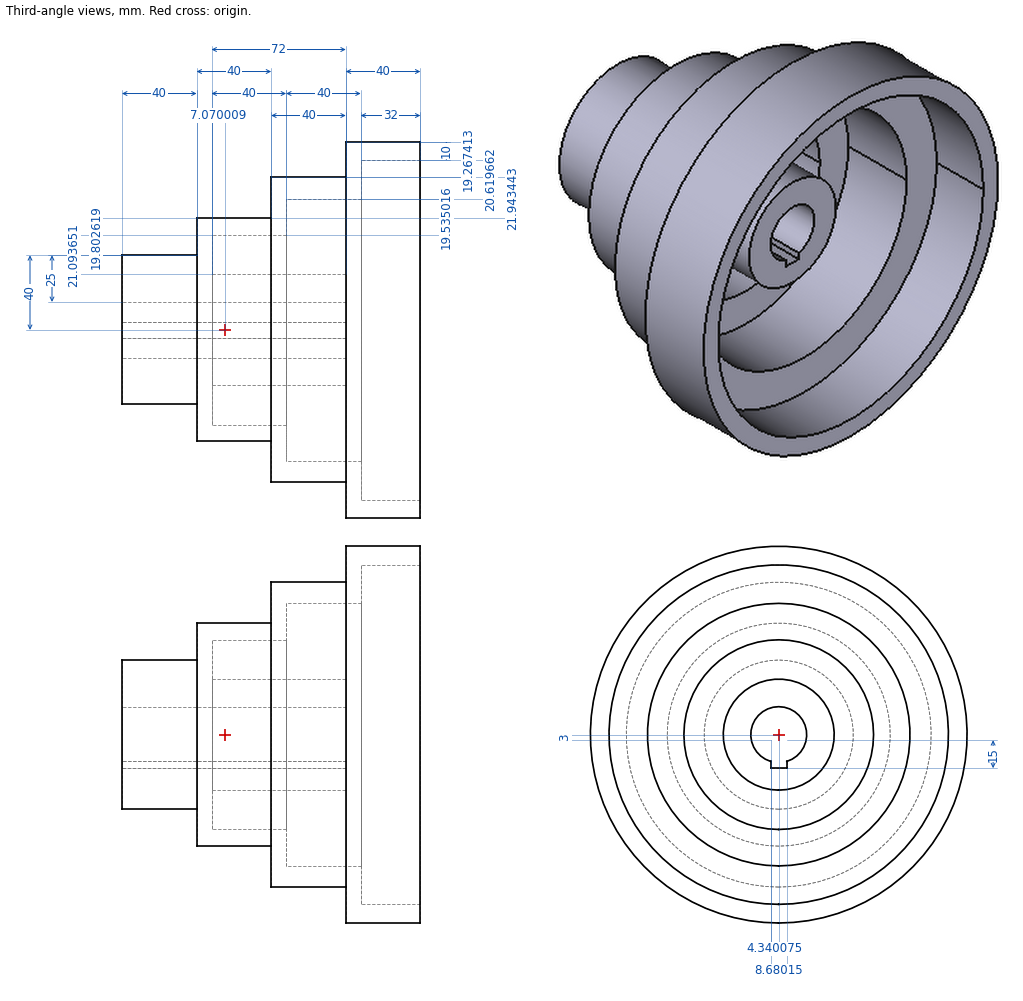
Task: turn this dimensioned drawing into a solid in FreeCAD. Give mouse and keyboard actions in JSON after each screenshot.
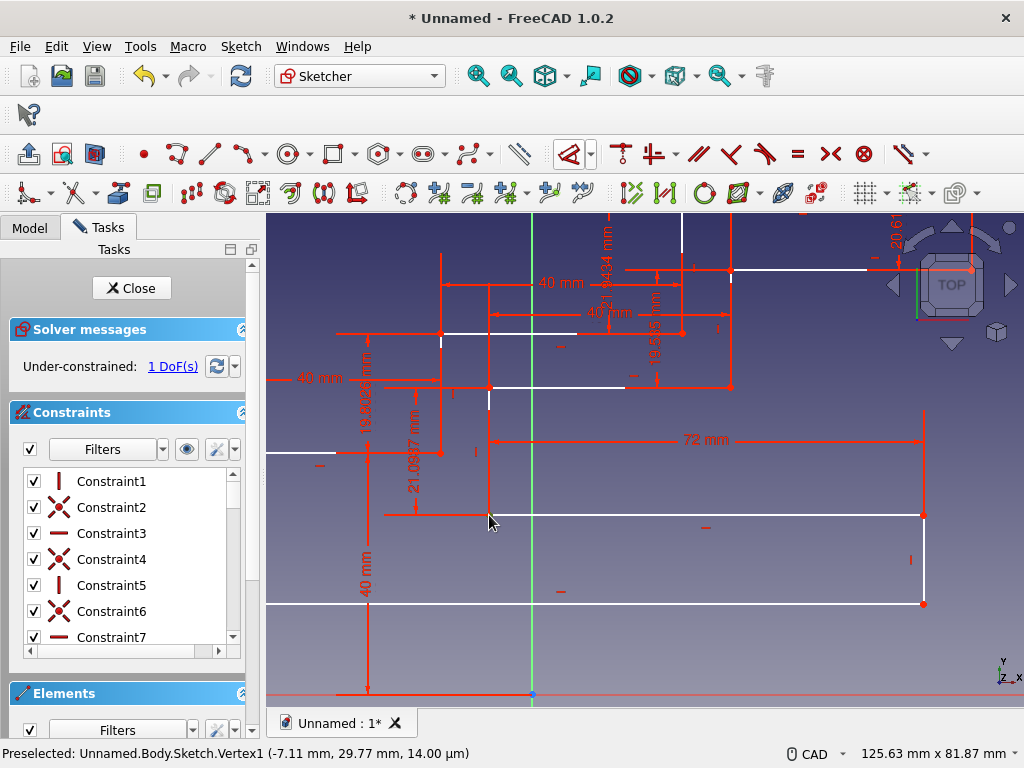
{"action": "key", "text": "l"}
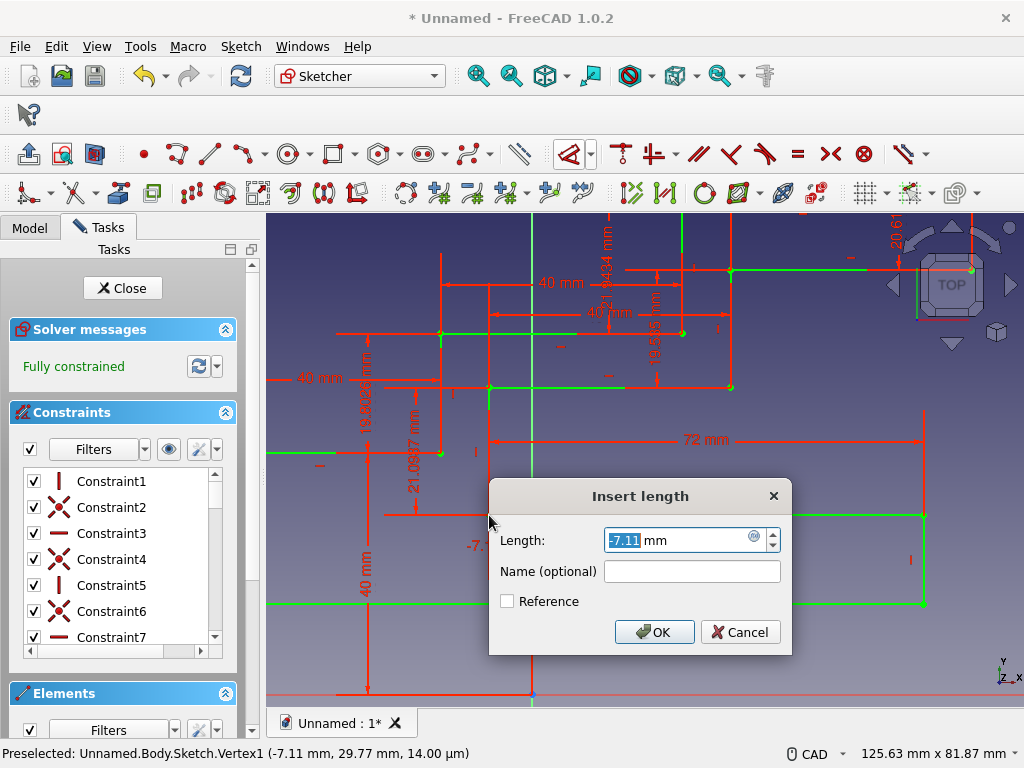
{"action": "type", "text": "-7.070009"}
{"action": "key", "text": "Return"}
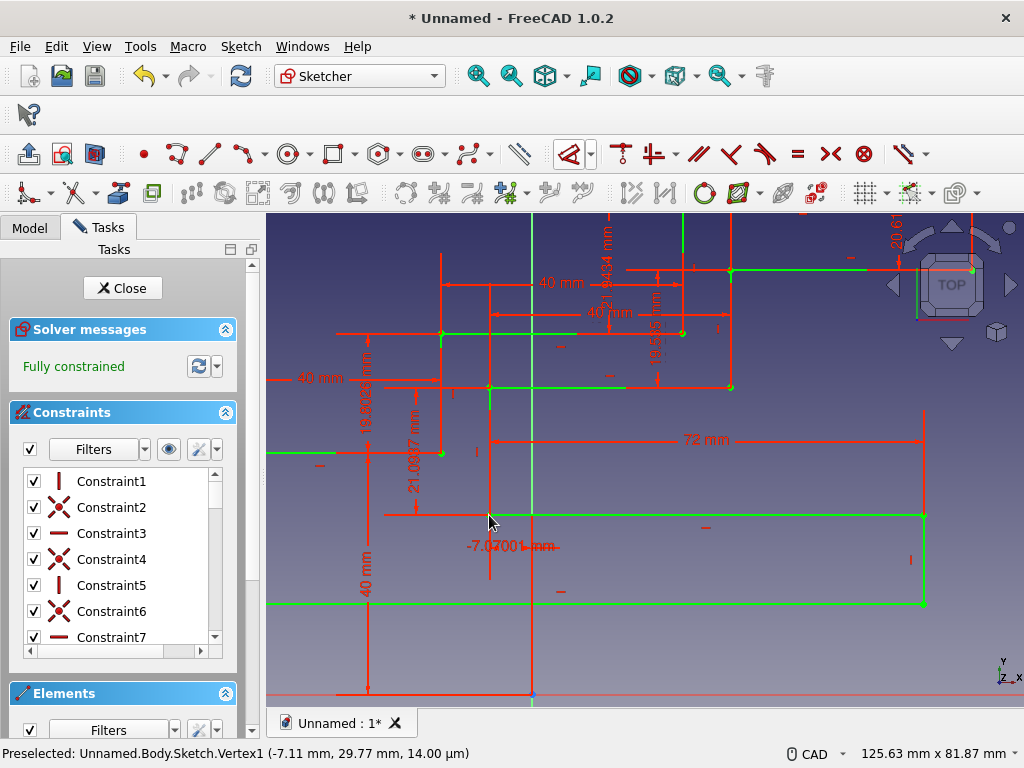
{"action": "left_click", "coordinate": [123, 288]}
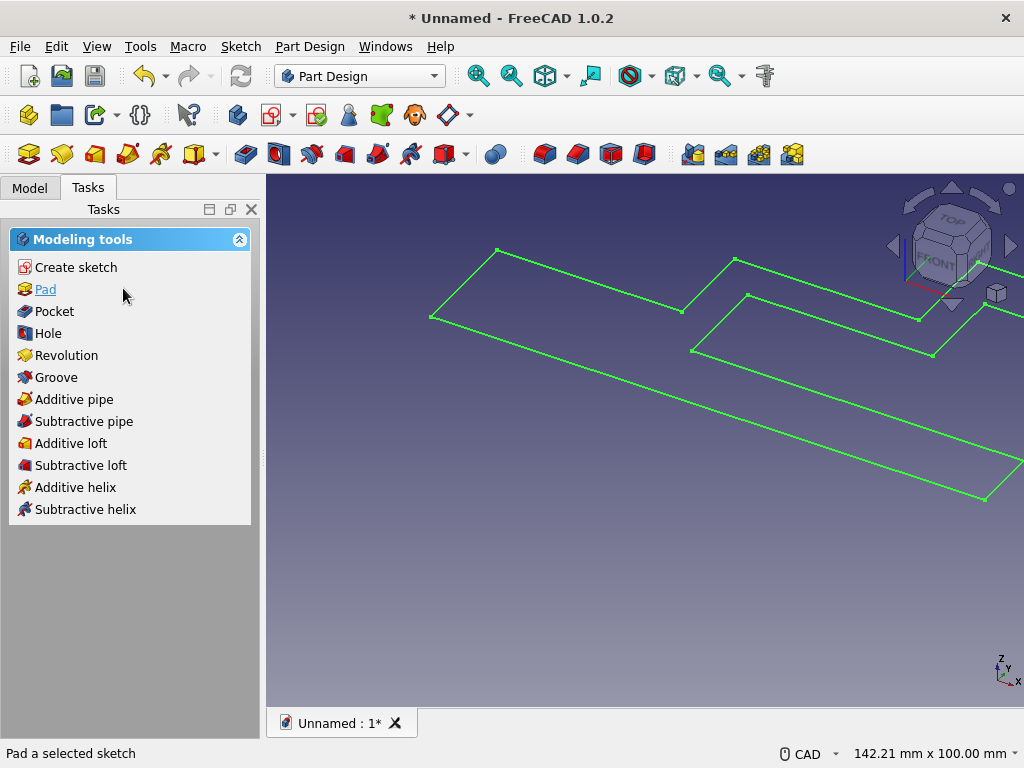
{"action": "left_click", "coordinate": [62, 154]}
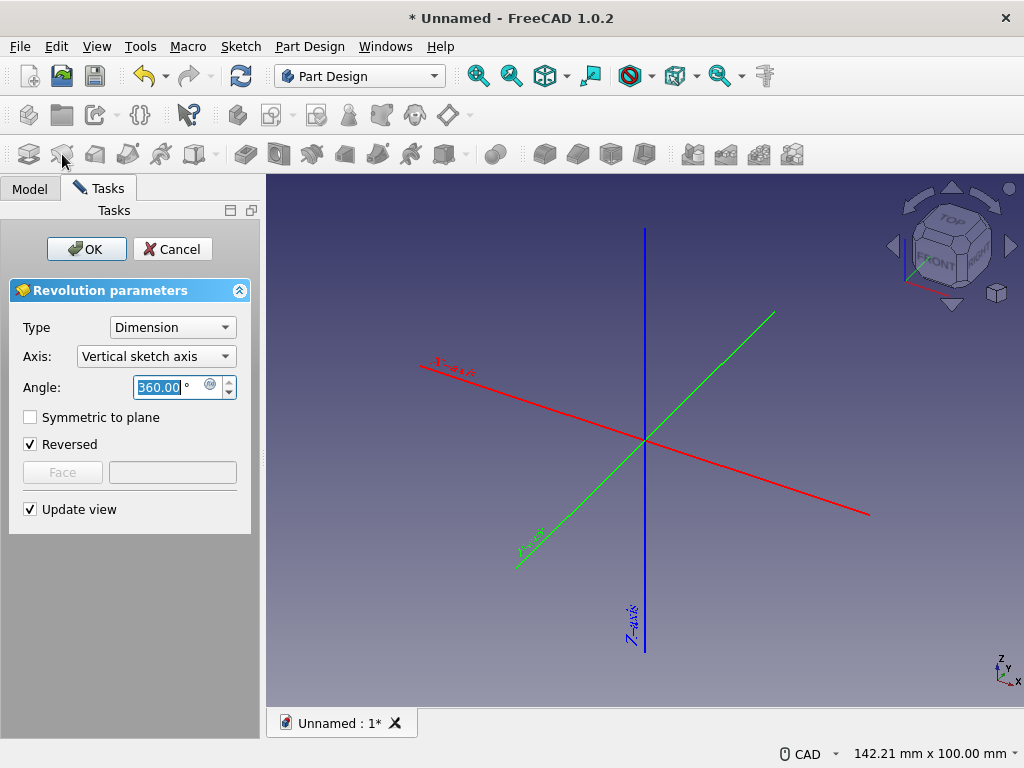
{"action": "left_click", "coordinate": [157, 356]}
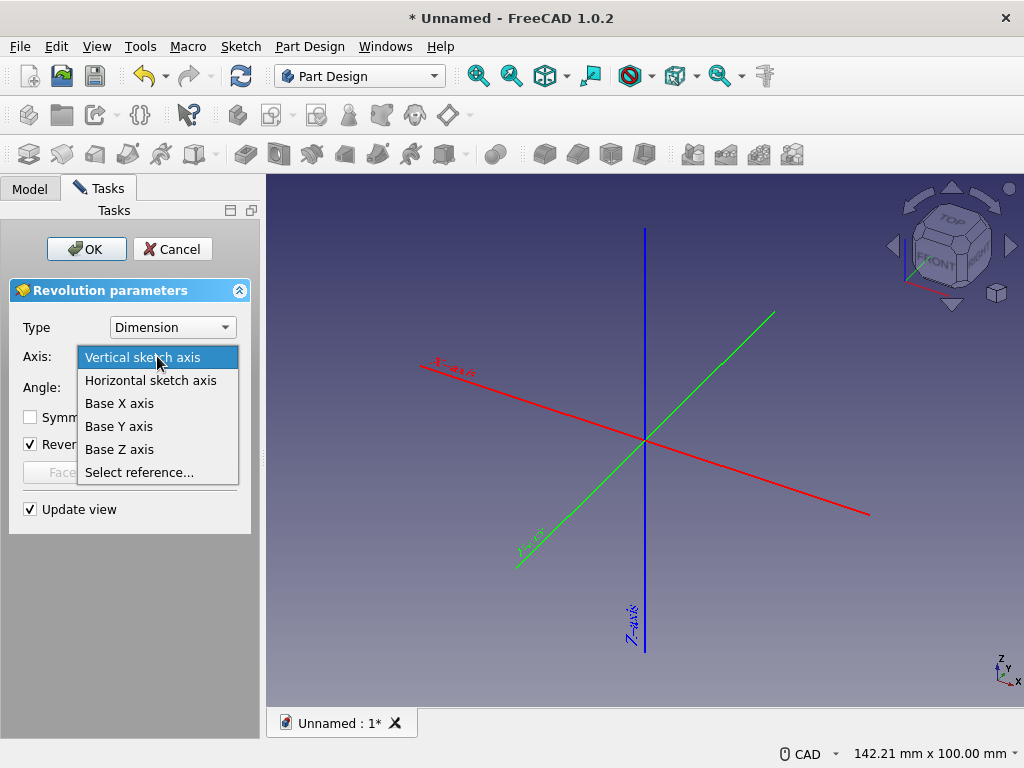
{"action": "left_click", "coordinate": [156, 380]}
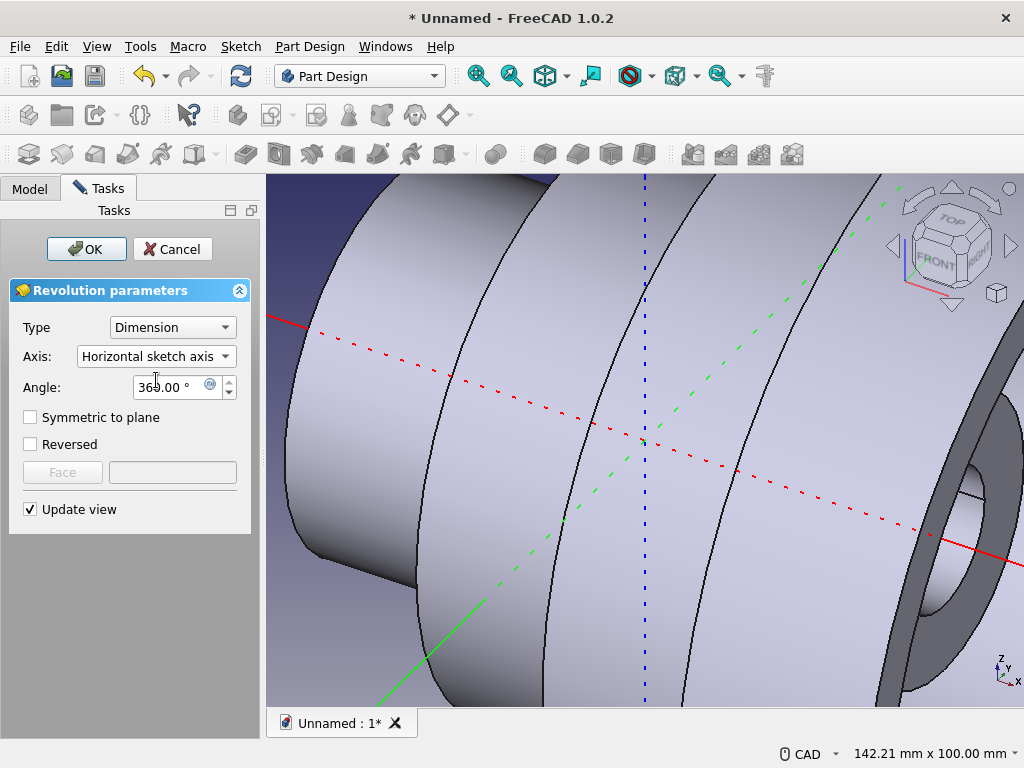
{"action": "left_click", "coordinate": [87, 249]}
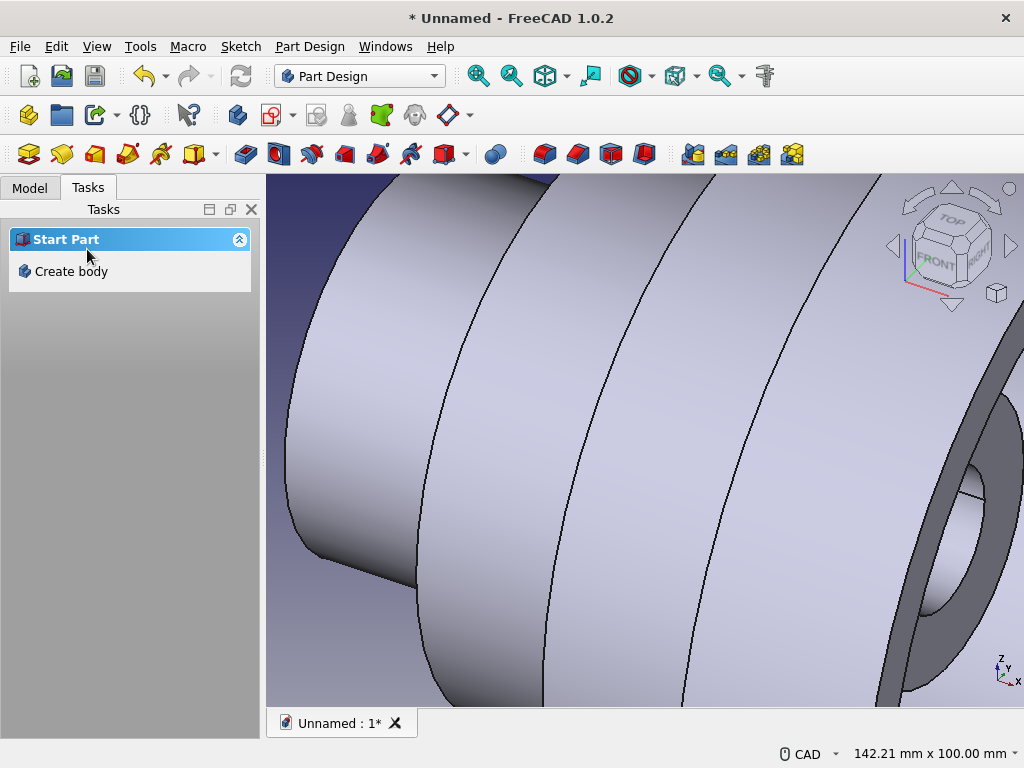
{"action": "left_click", "coordinate": [479, 76]}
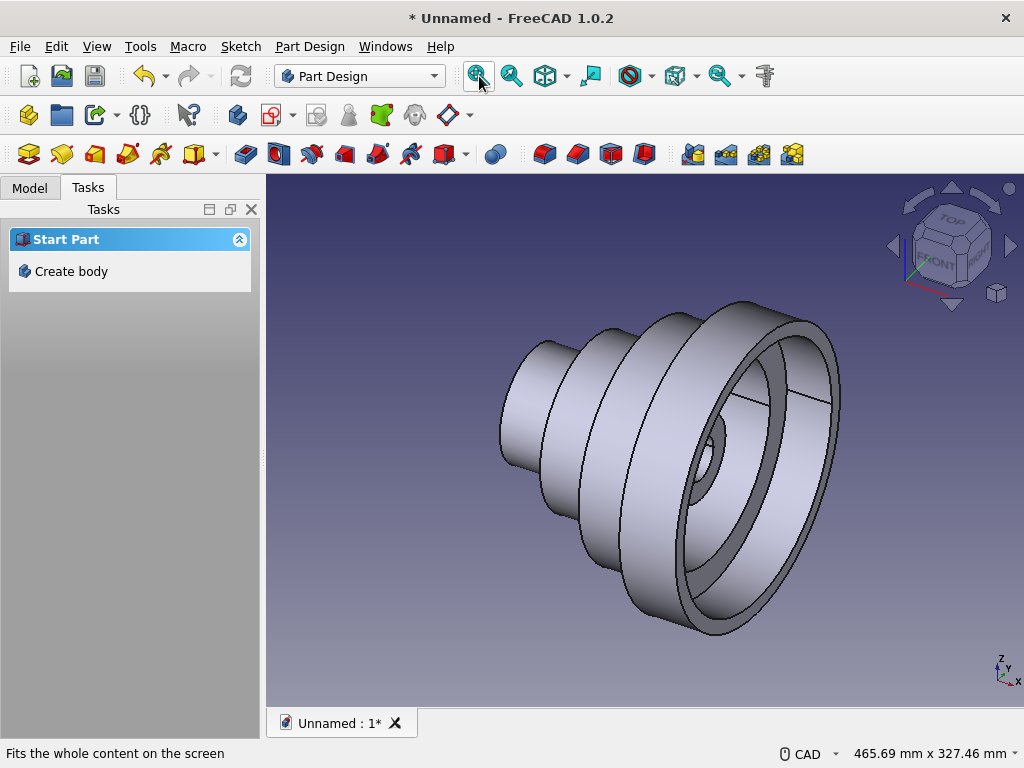
{"action": "left_click", "coordinate": [270, 116]}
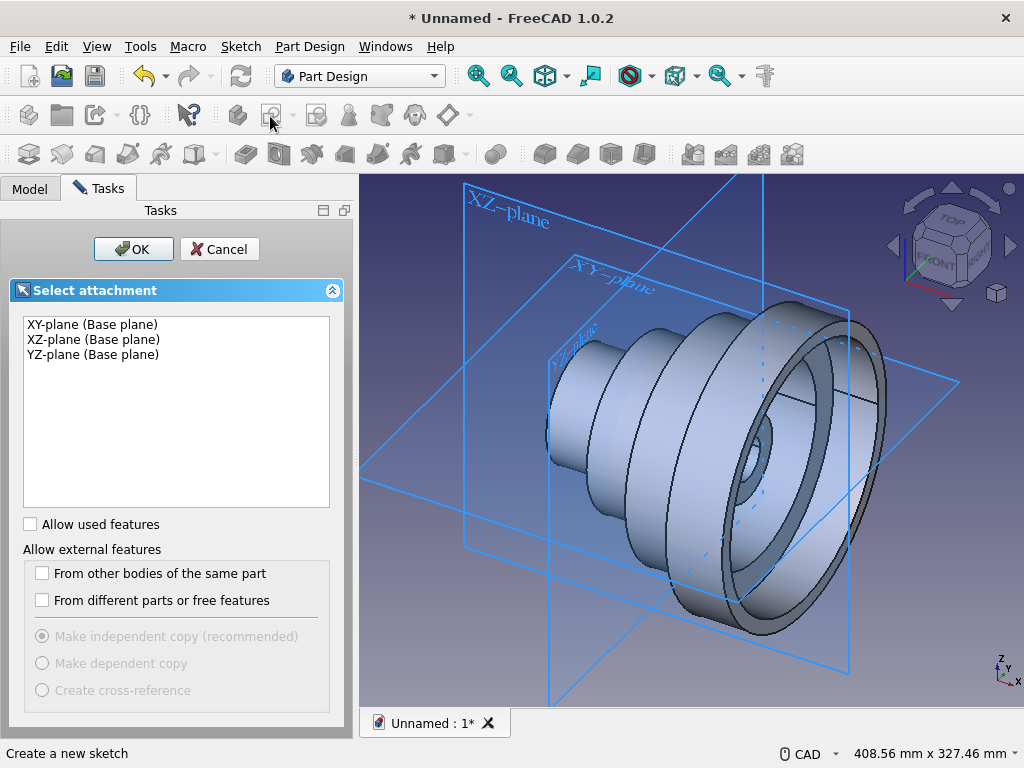
{"action": "left_click", "coordinate": [84, 354]}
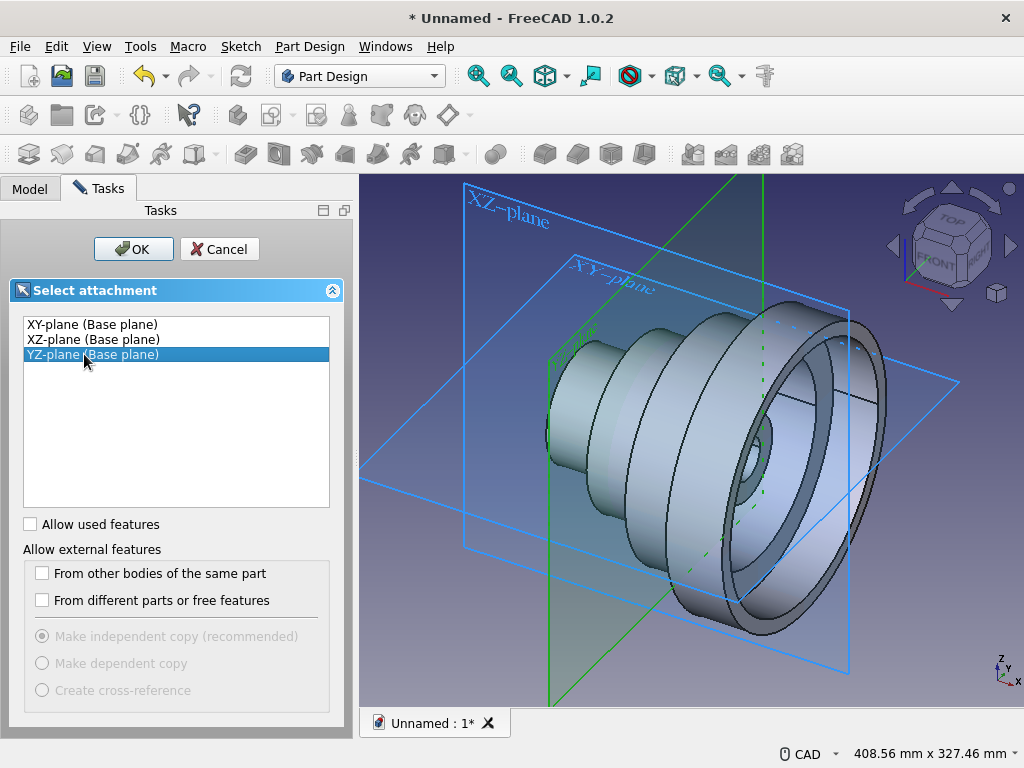
{"action": "left_click", "coordinate": [134, 249]}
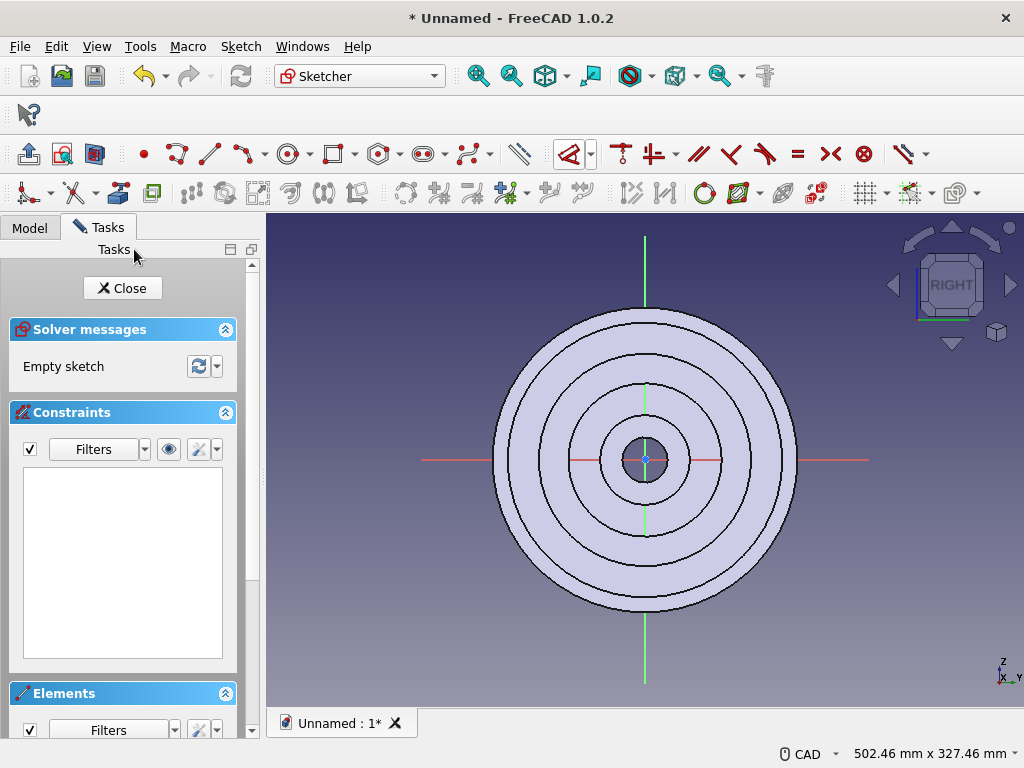
{"action": "left_click", "coordinate": [95, 154]}